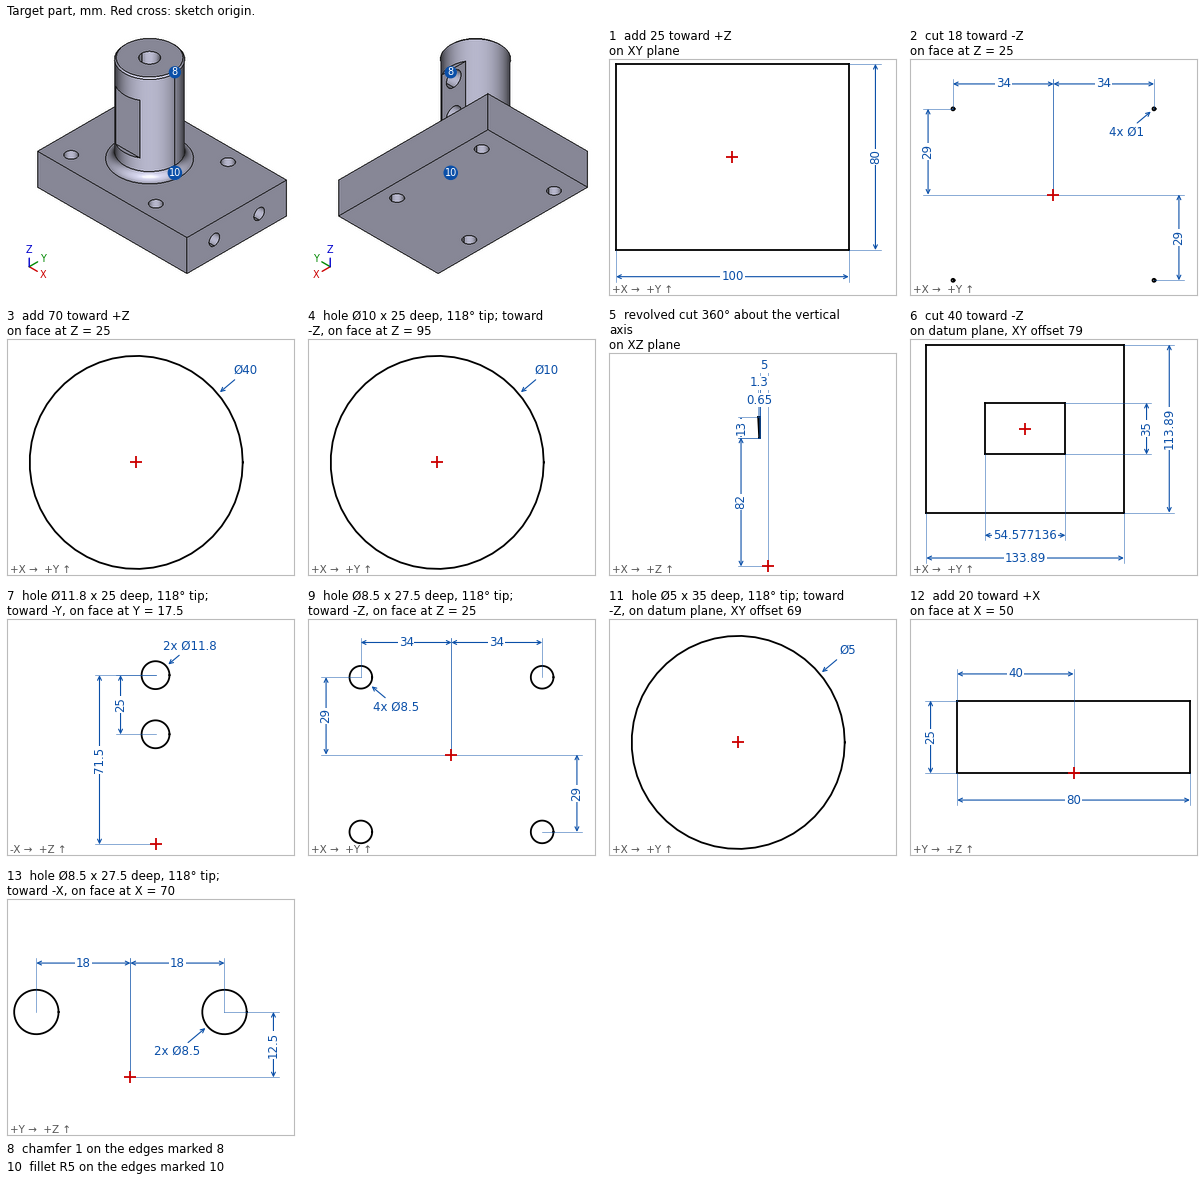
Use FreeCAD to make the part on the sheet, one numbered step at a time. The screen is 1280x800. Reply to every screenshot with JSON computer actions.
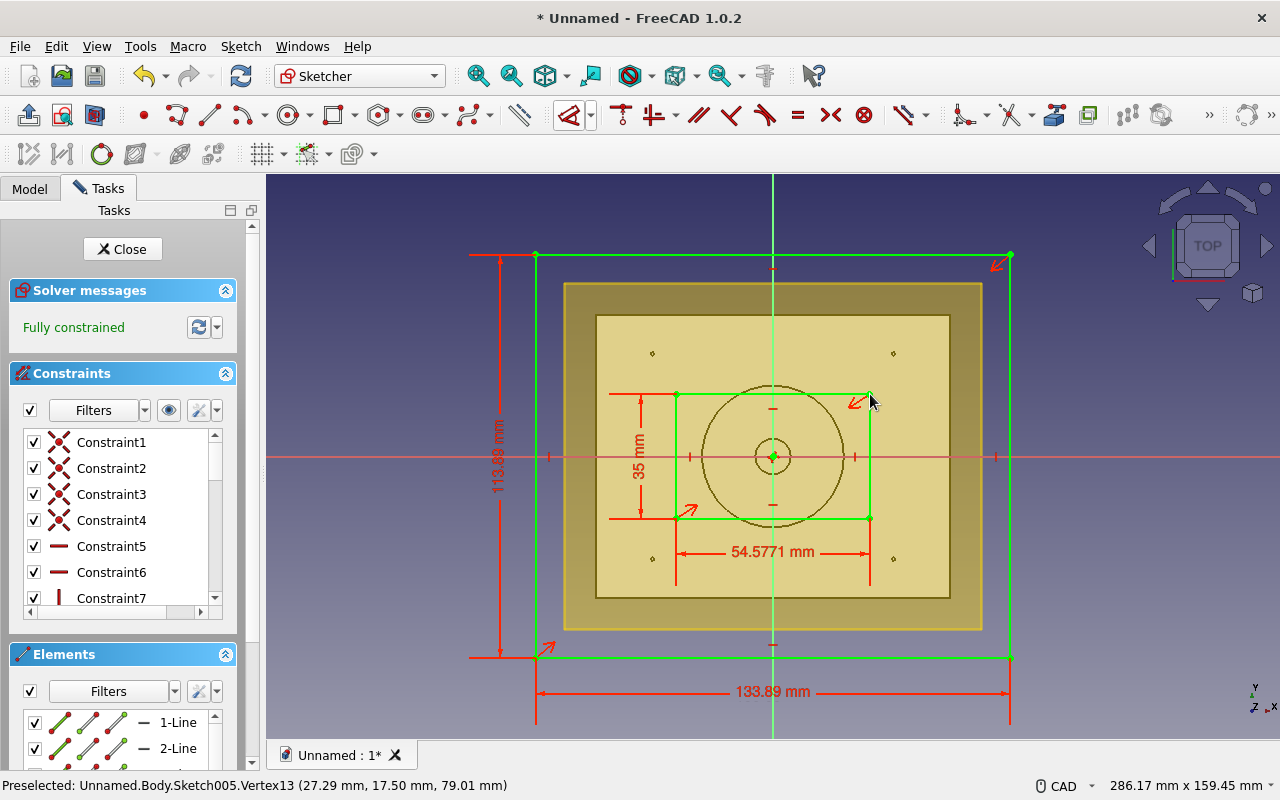
{"action": "left_click", "coordinate": [123, 249]}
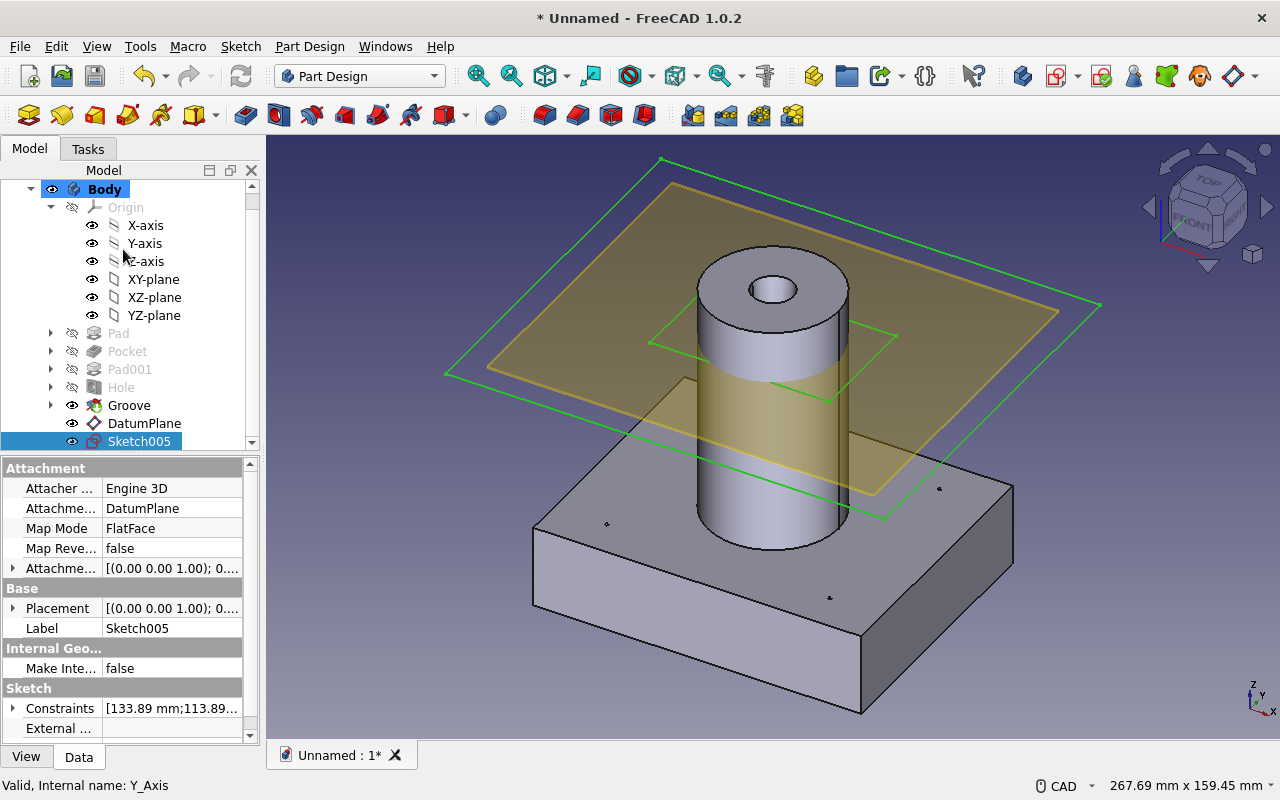
{"action": "left_click", "coordinate": [246, 116]}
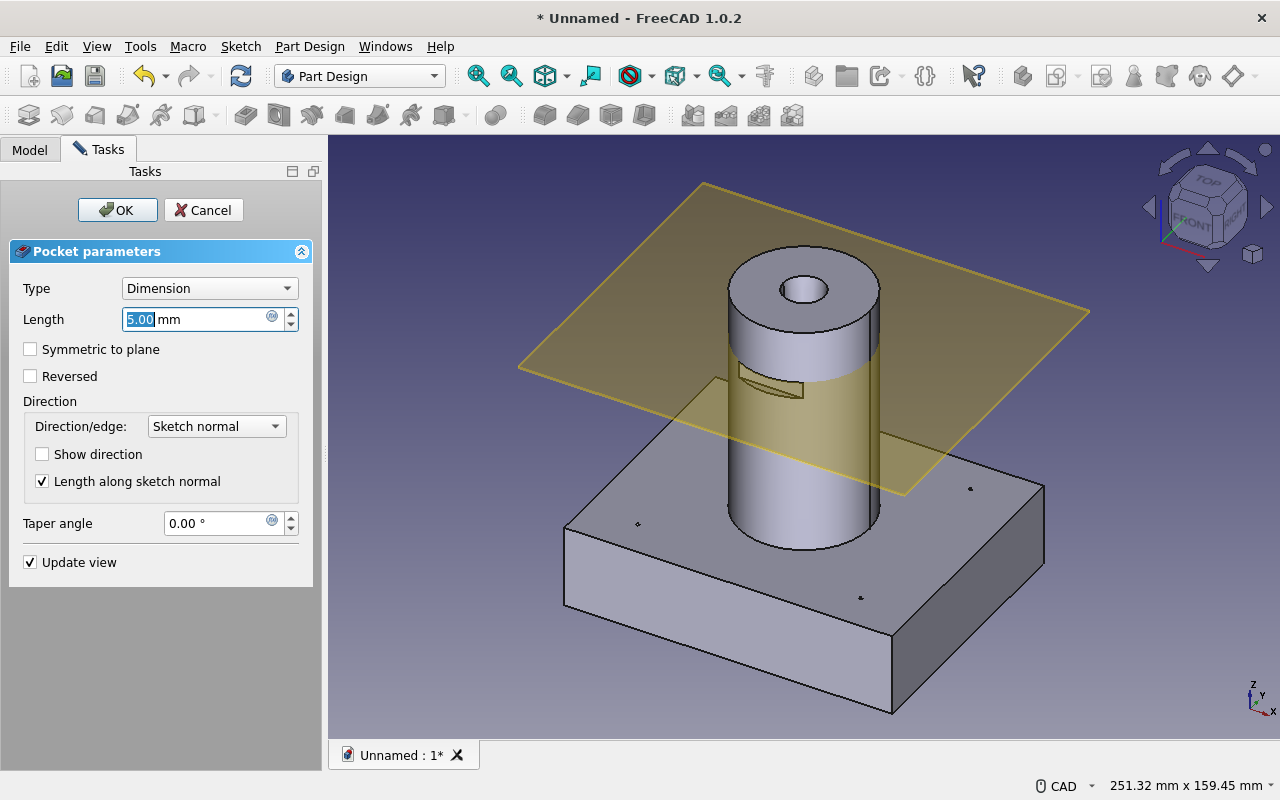
{"action": "type", "text": "40"}
{"action": "key", "text": "Tab"}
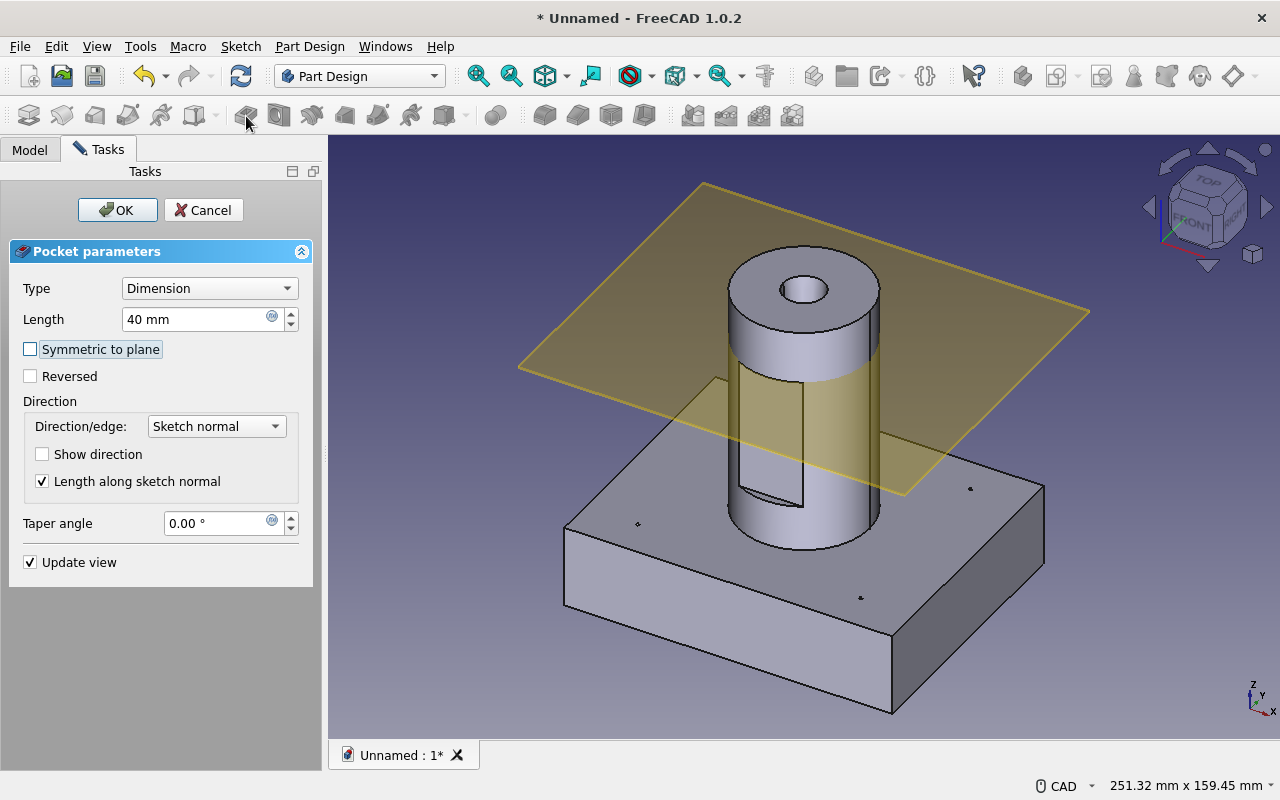
{"action": "left_click", "coordinate": [118, 210]}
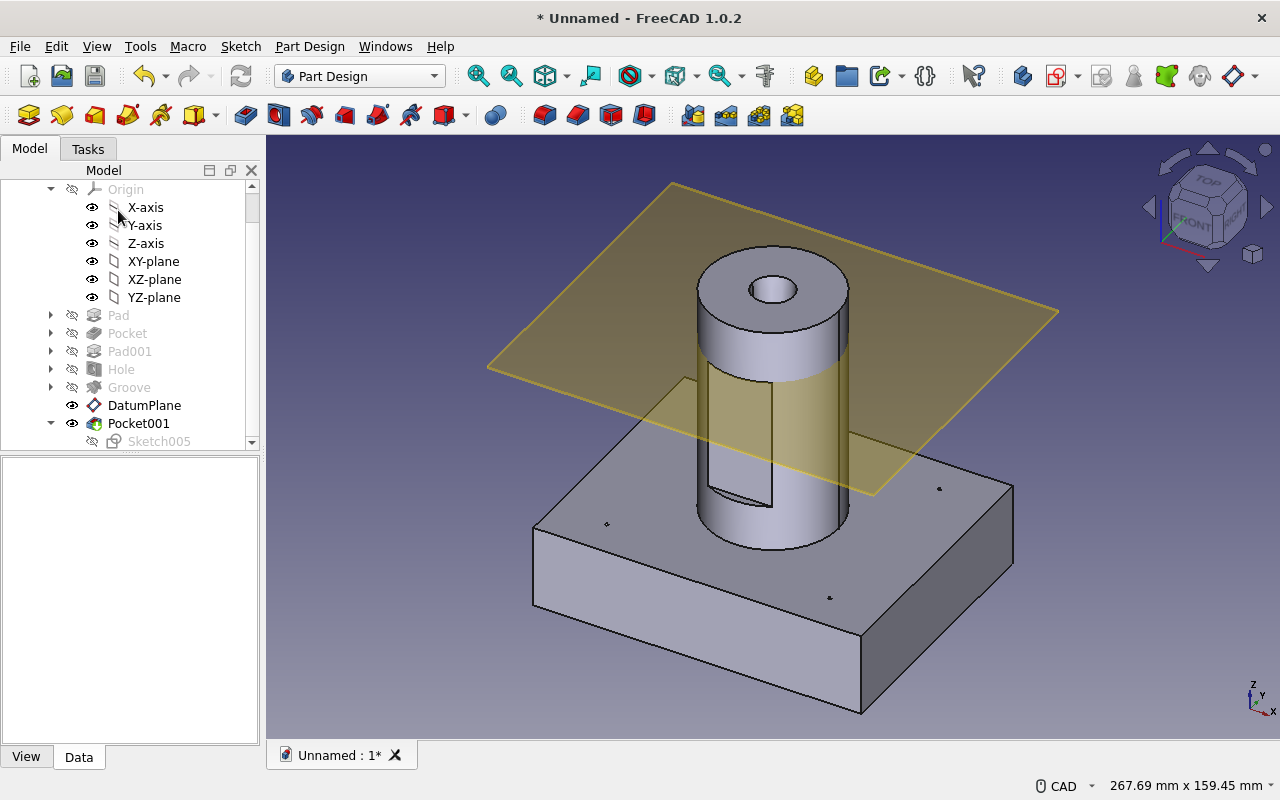
{"action": "left_click", "coordinate": [117, 405]}
{"action": "key", "text": "space"}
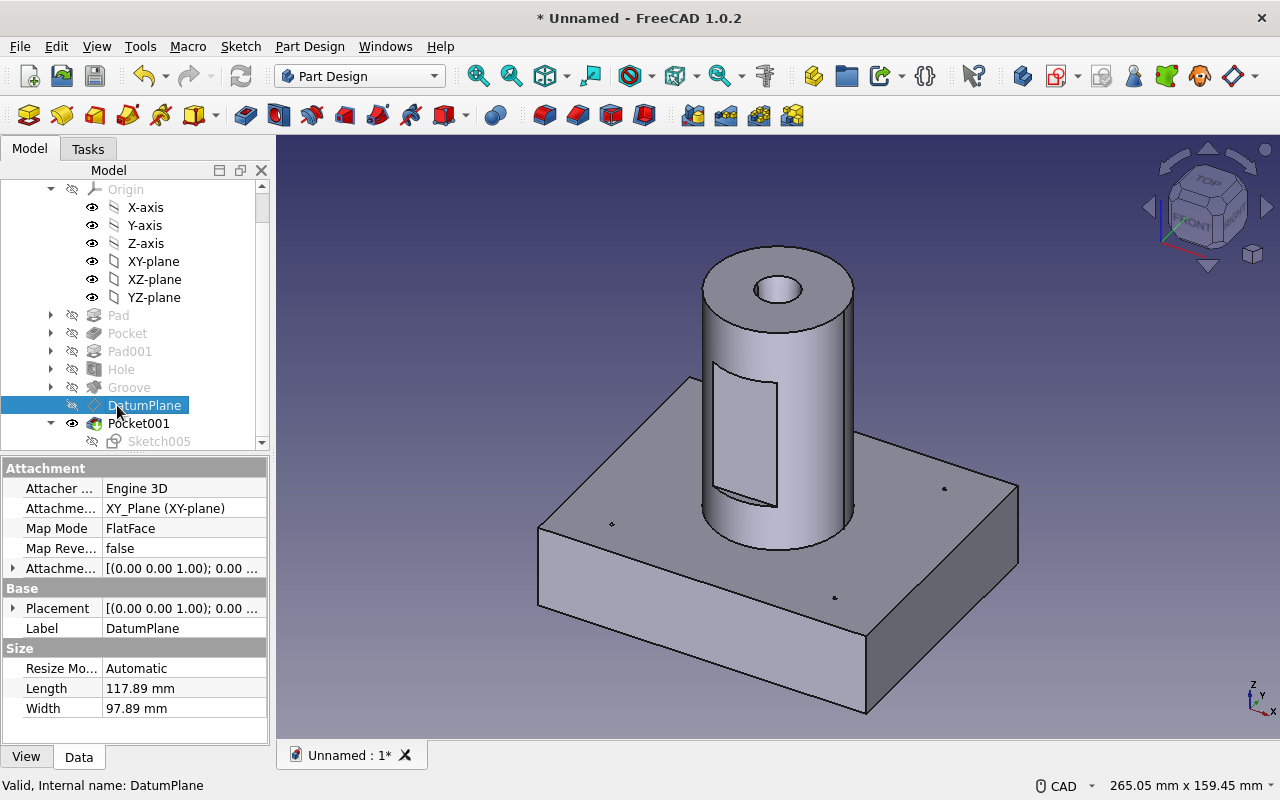
{"action": "key", "text": "4"}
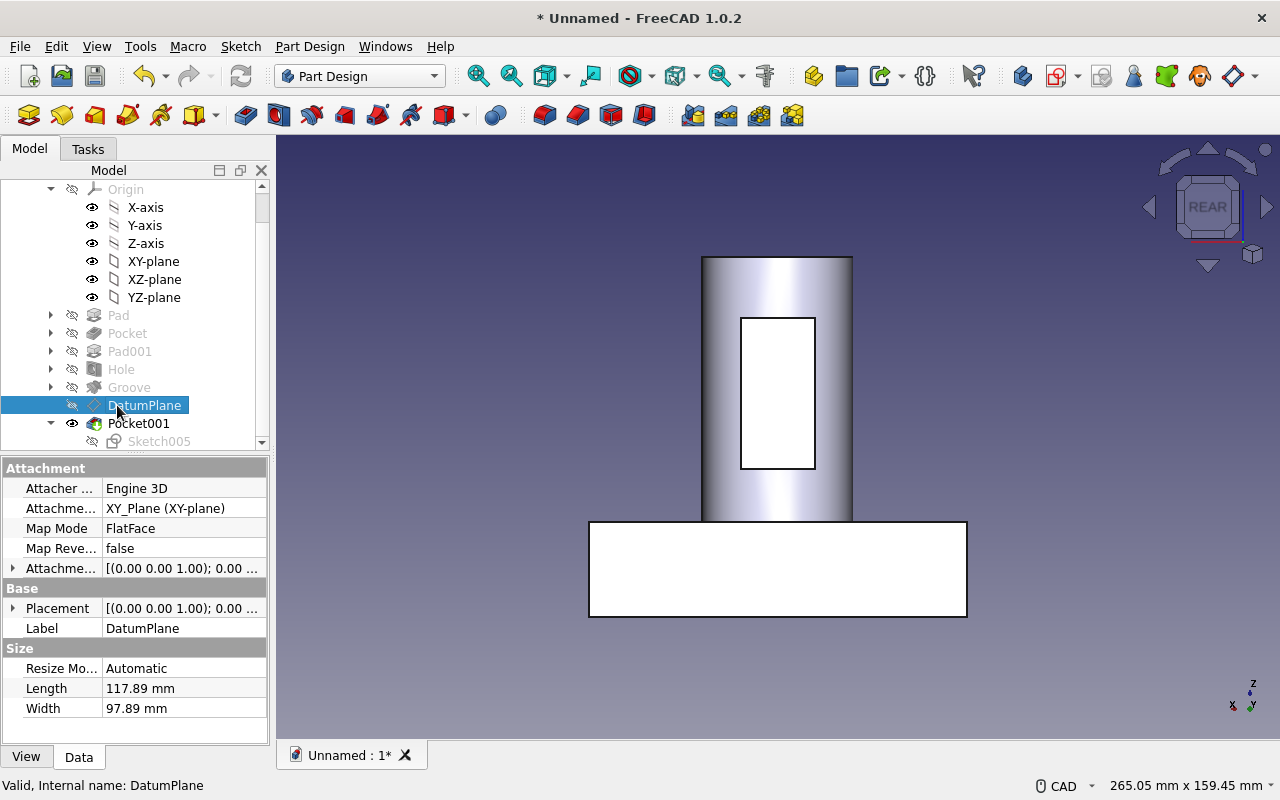
{"action": "left_click", "coordinate": [778, 371]}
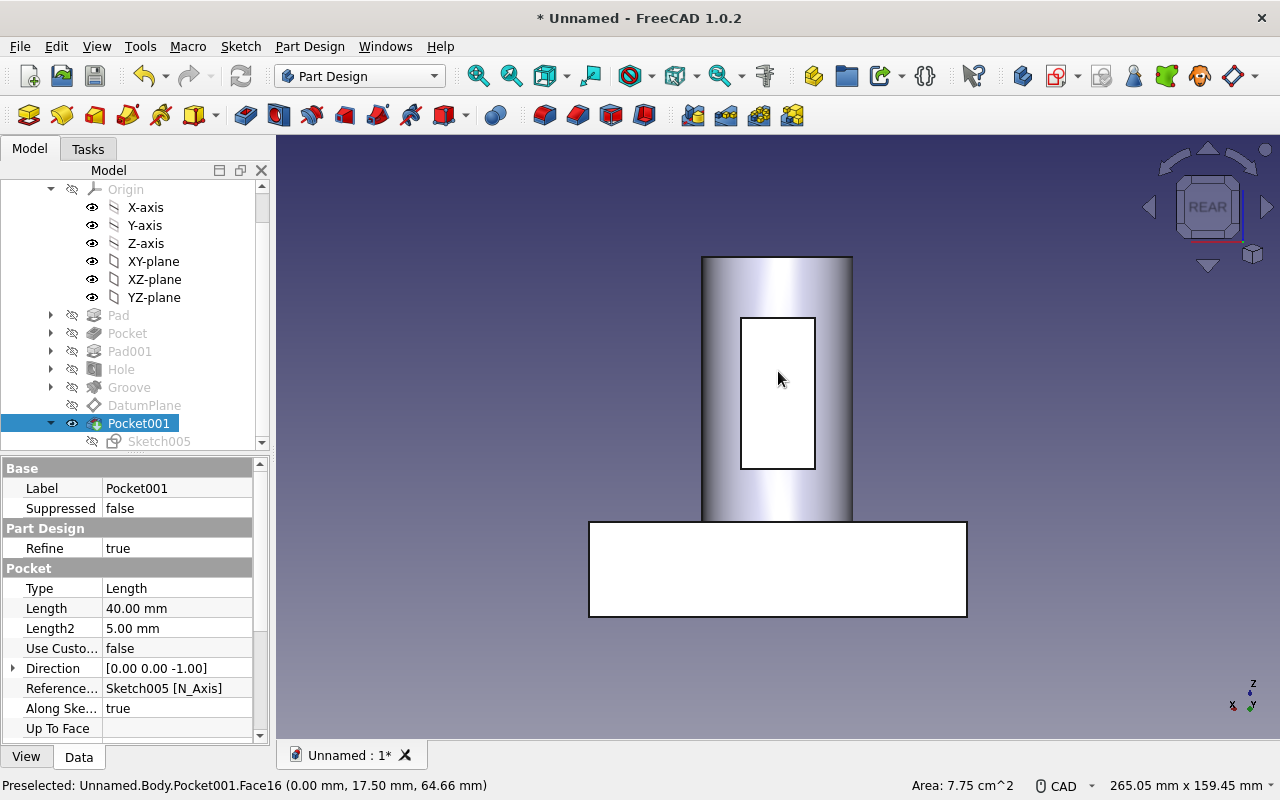
{"action": "left_click", "coordinate": [1056, 76]}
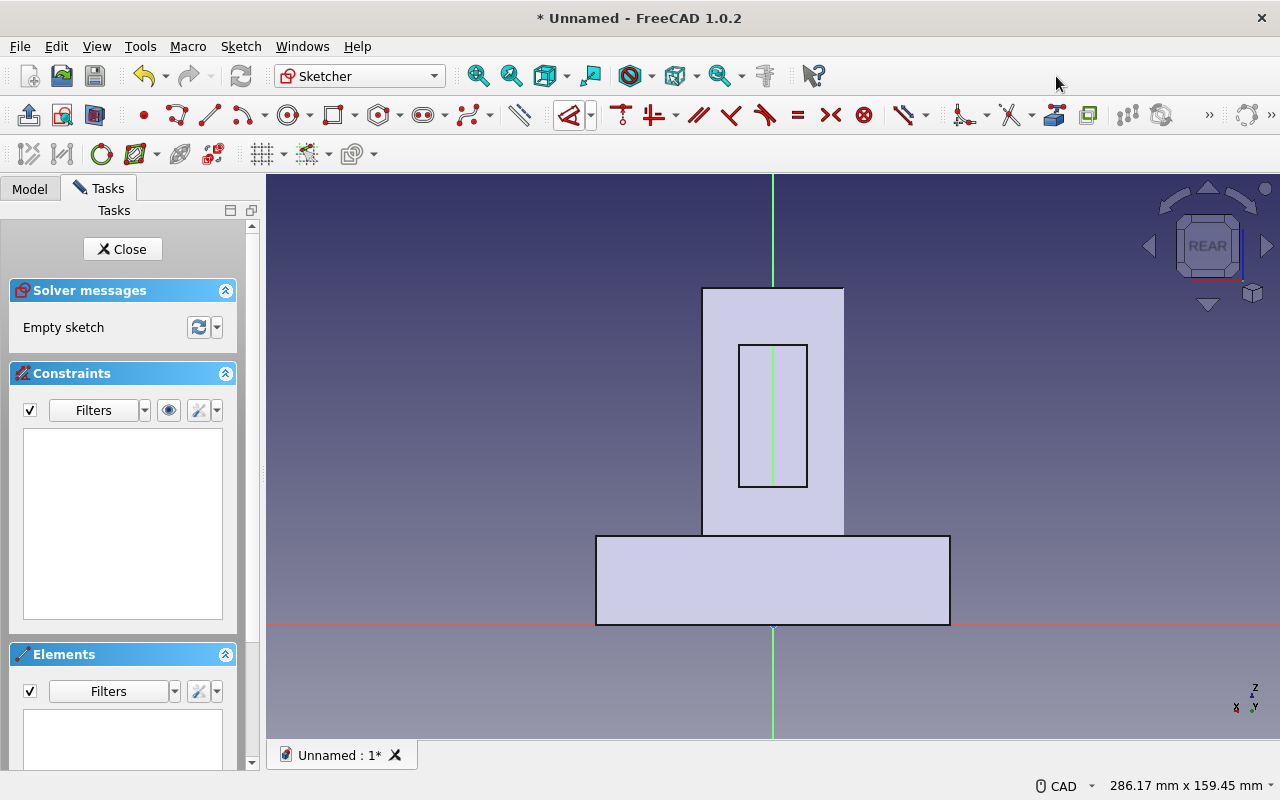
{"action": "key", "text": "q s"}